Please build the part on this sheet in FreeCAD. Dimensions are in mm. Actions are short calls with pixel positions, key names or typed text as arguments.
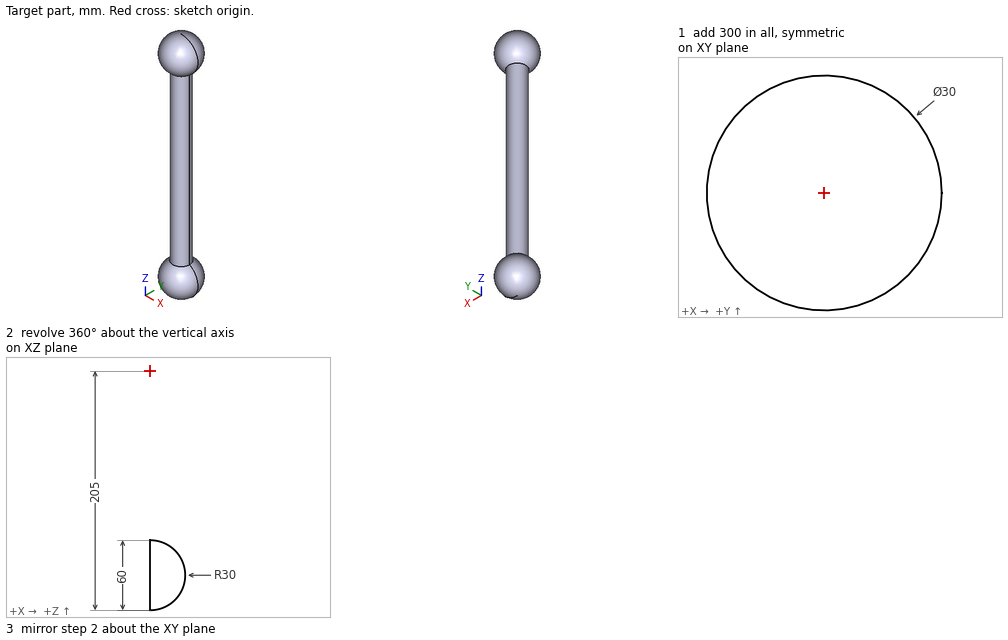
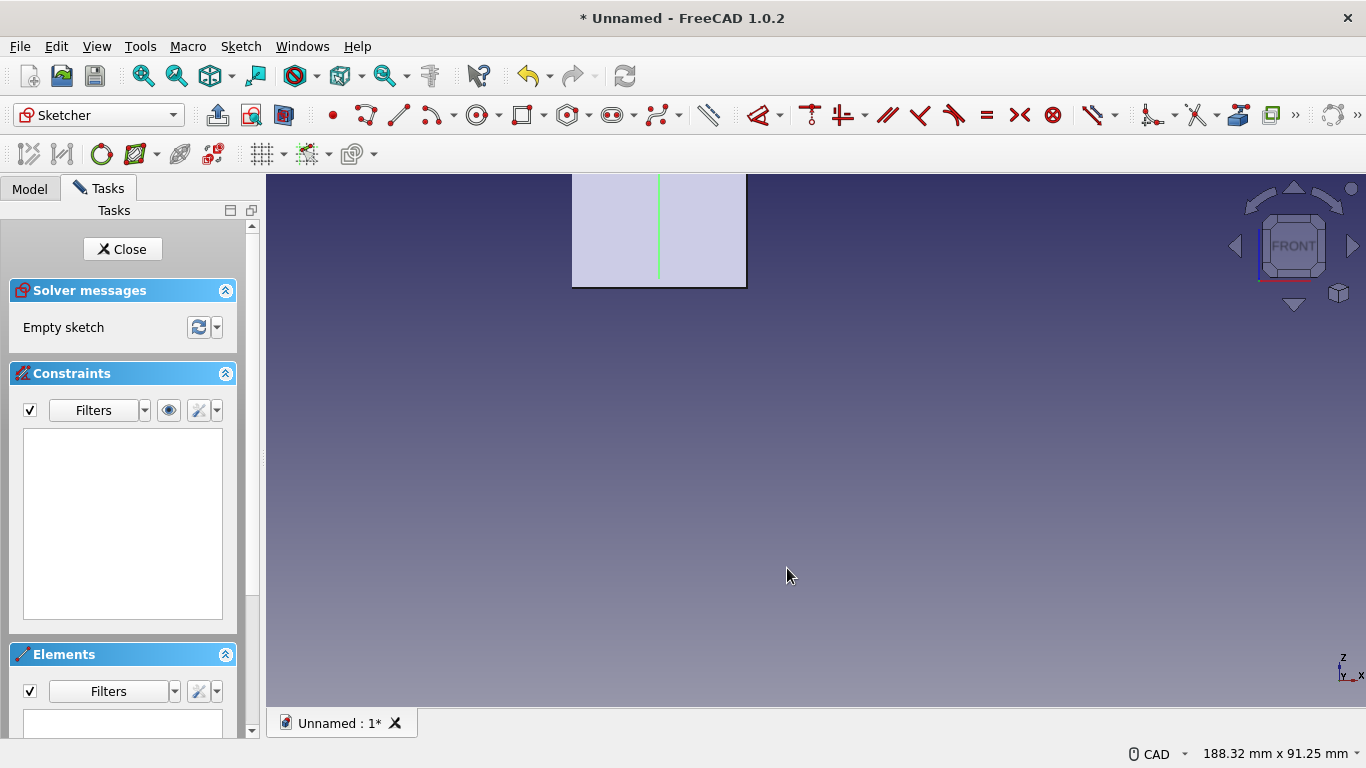
click(399, 116)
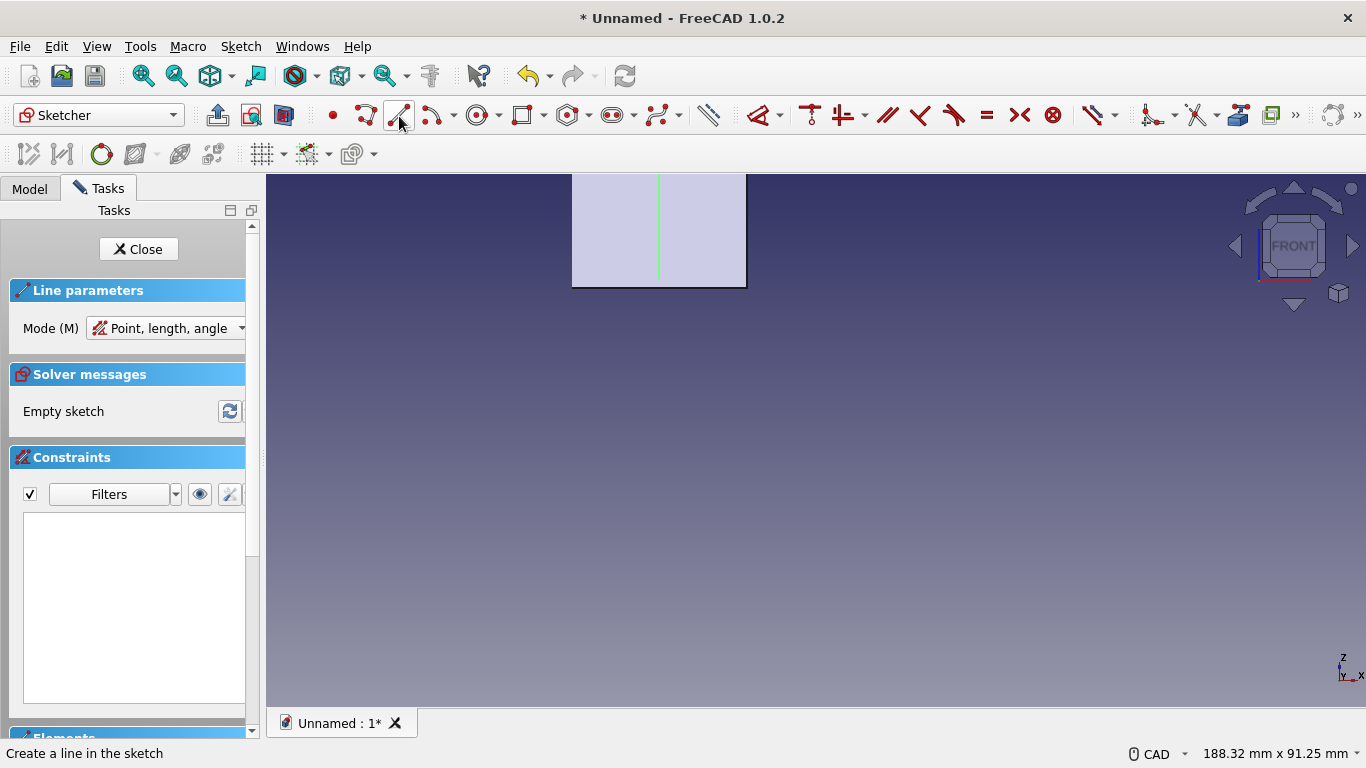
click(659, 609)
click(668, 258)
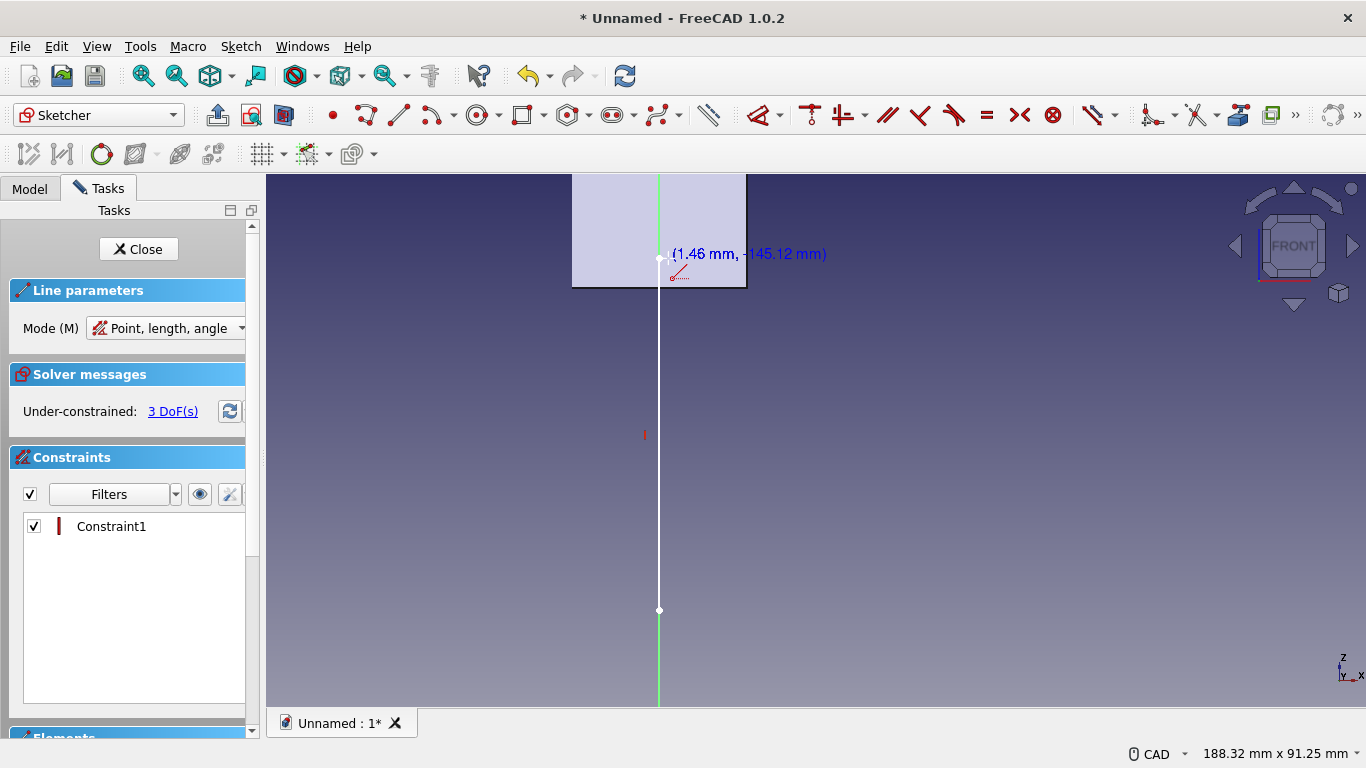
click(454, 116)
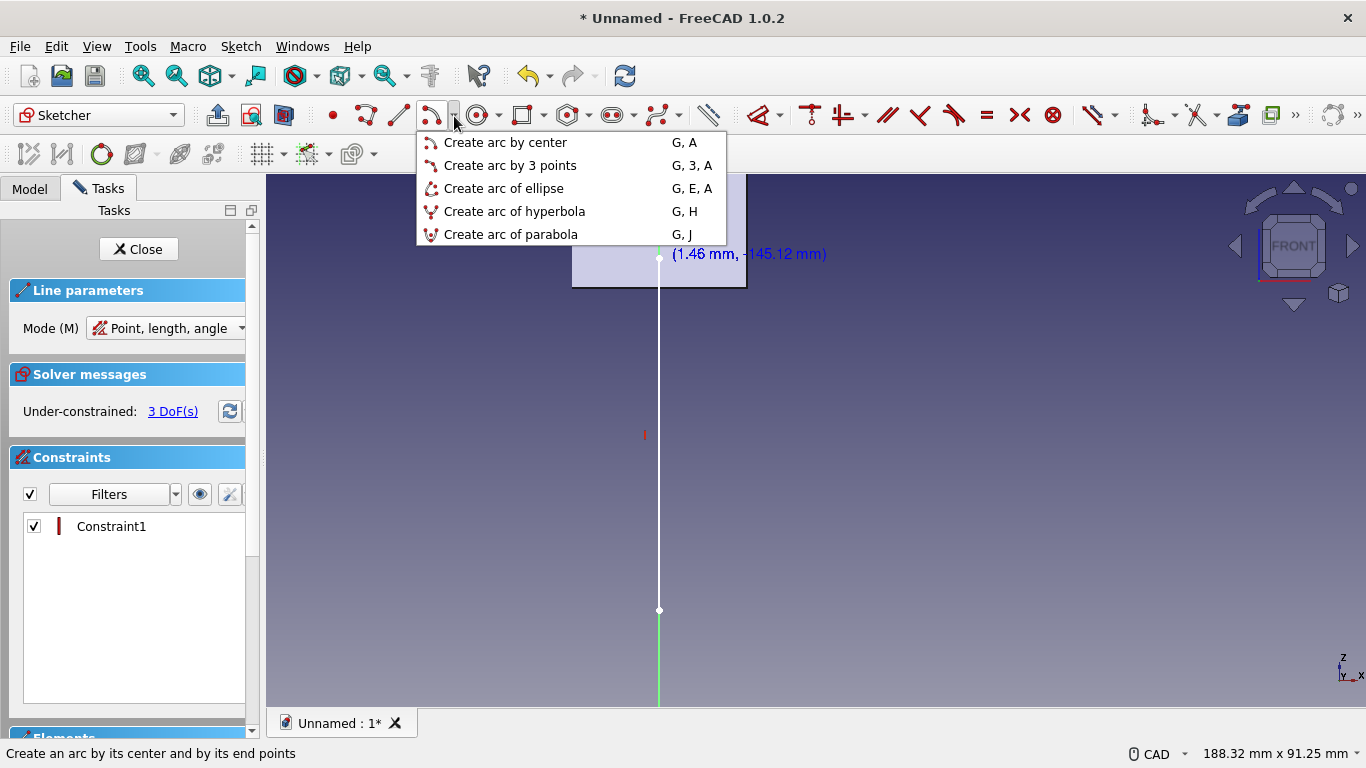
click(572, 166)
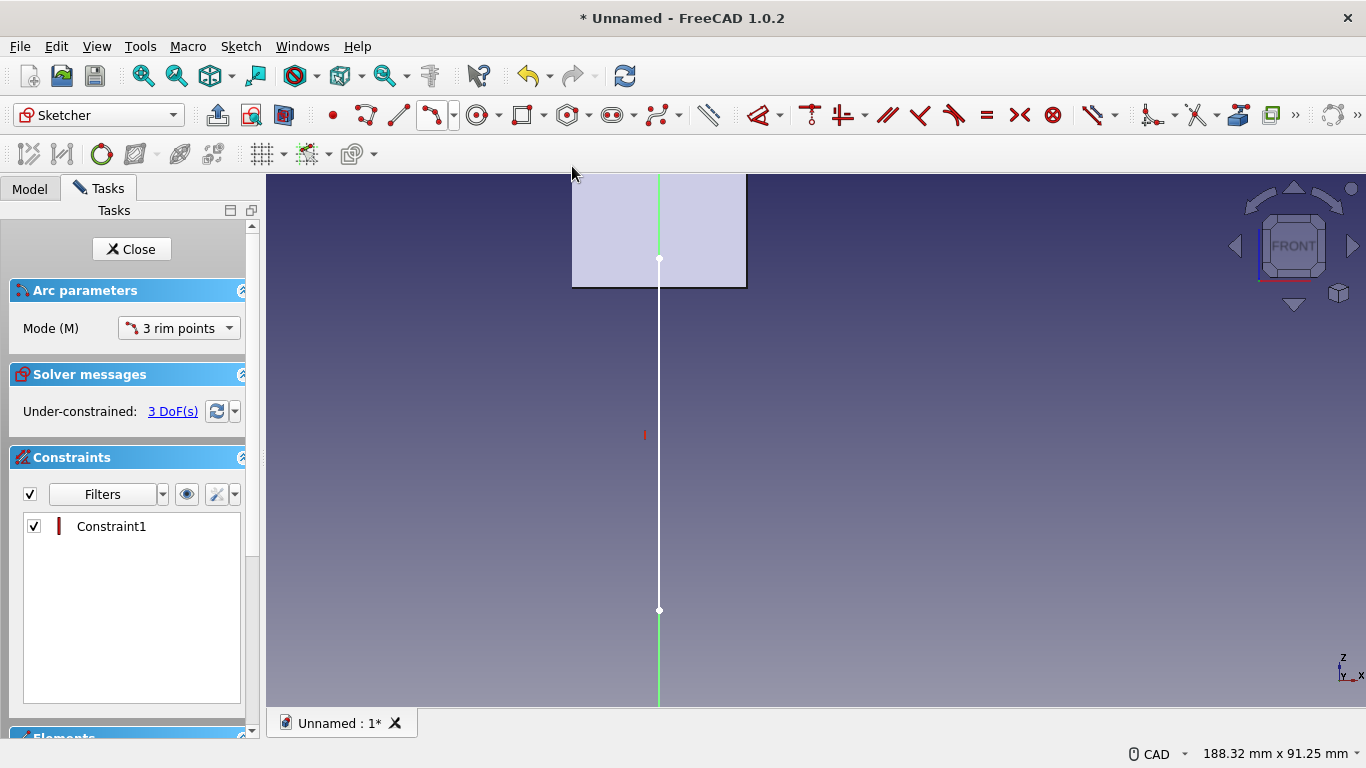
click(668, 258)
click(659, 610)
click(835, 434)
key(Escape)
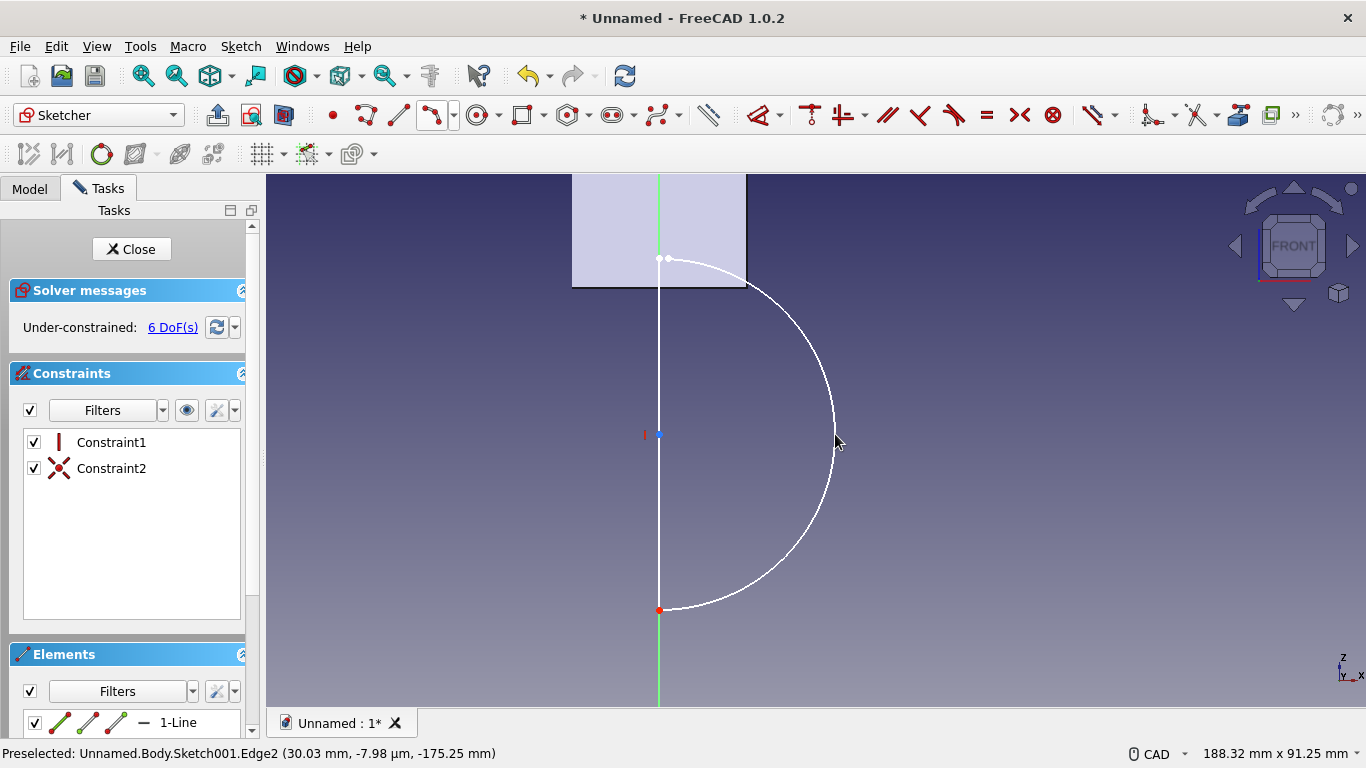
click(659, 434)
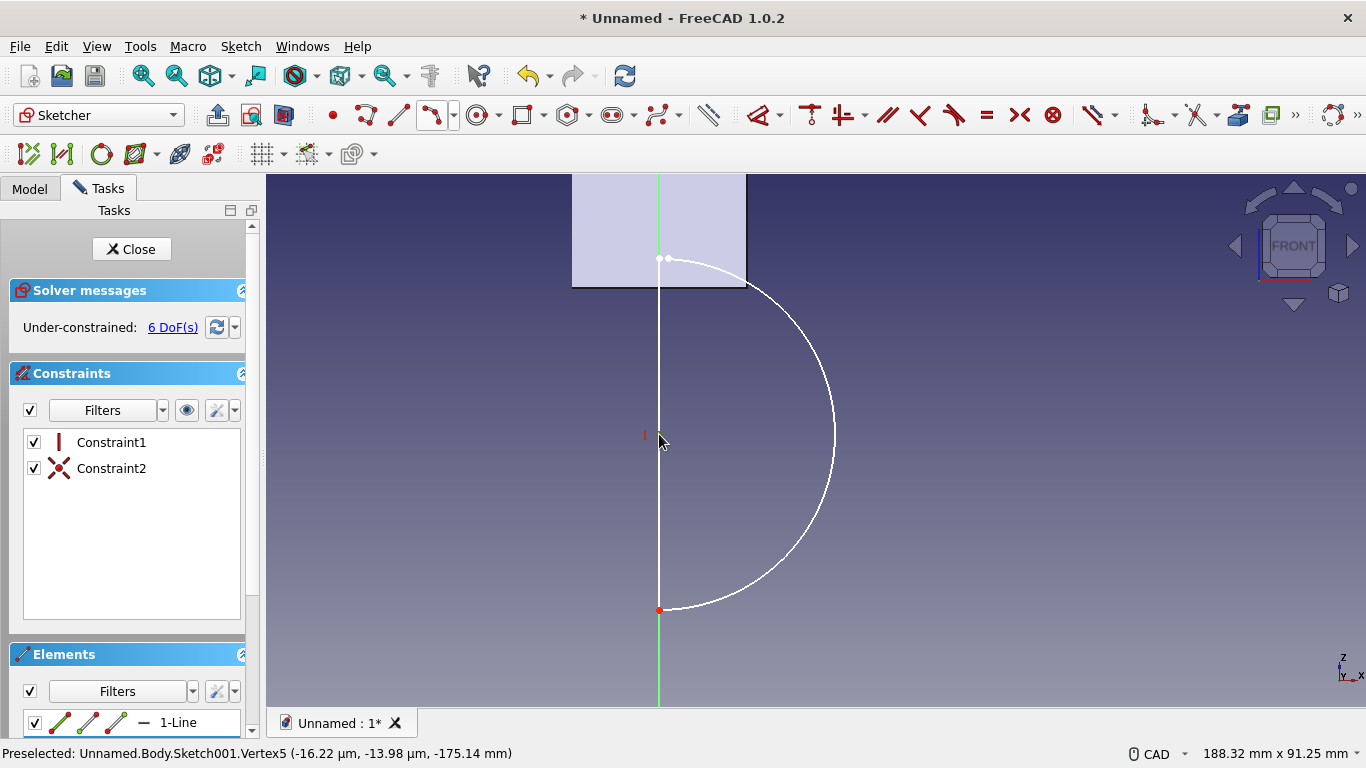
click(659, 645)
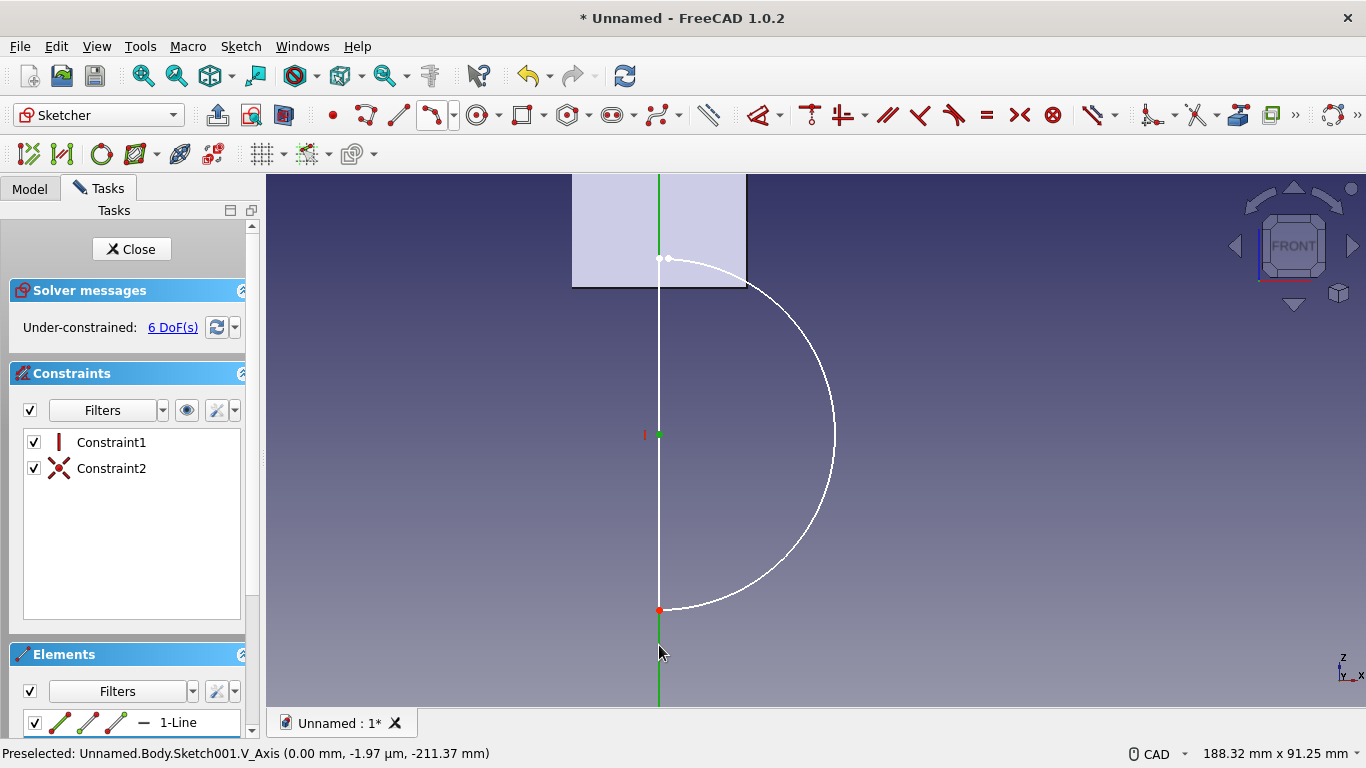
click(810, 116)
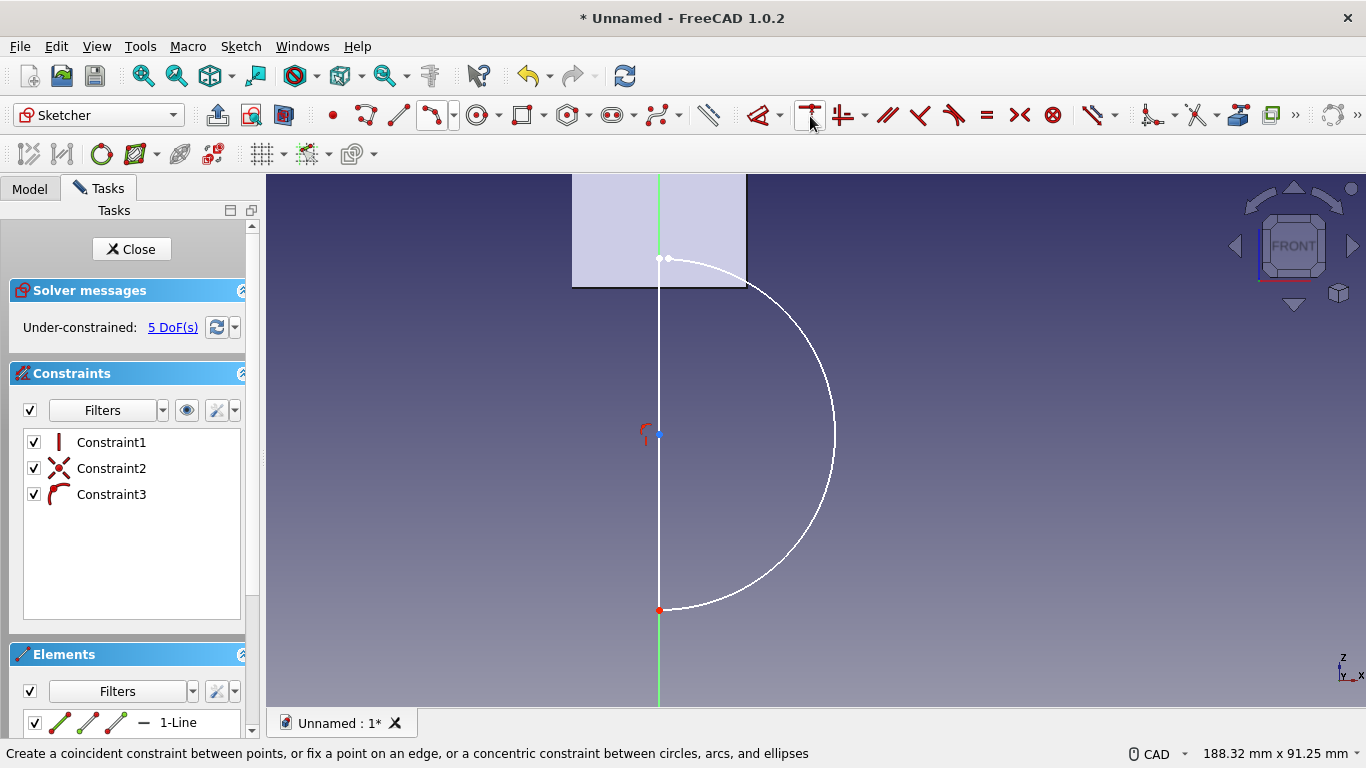
click(800, 540)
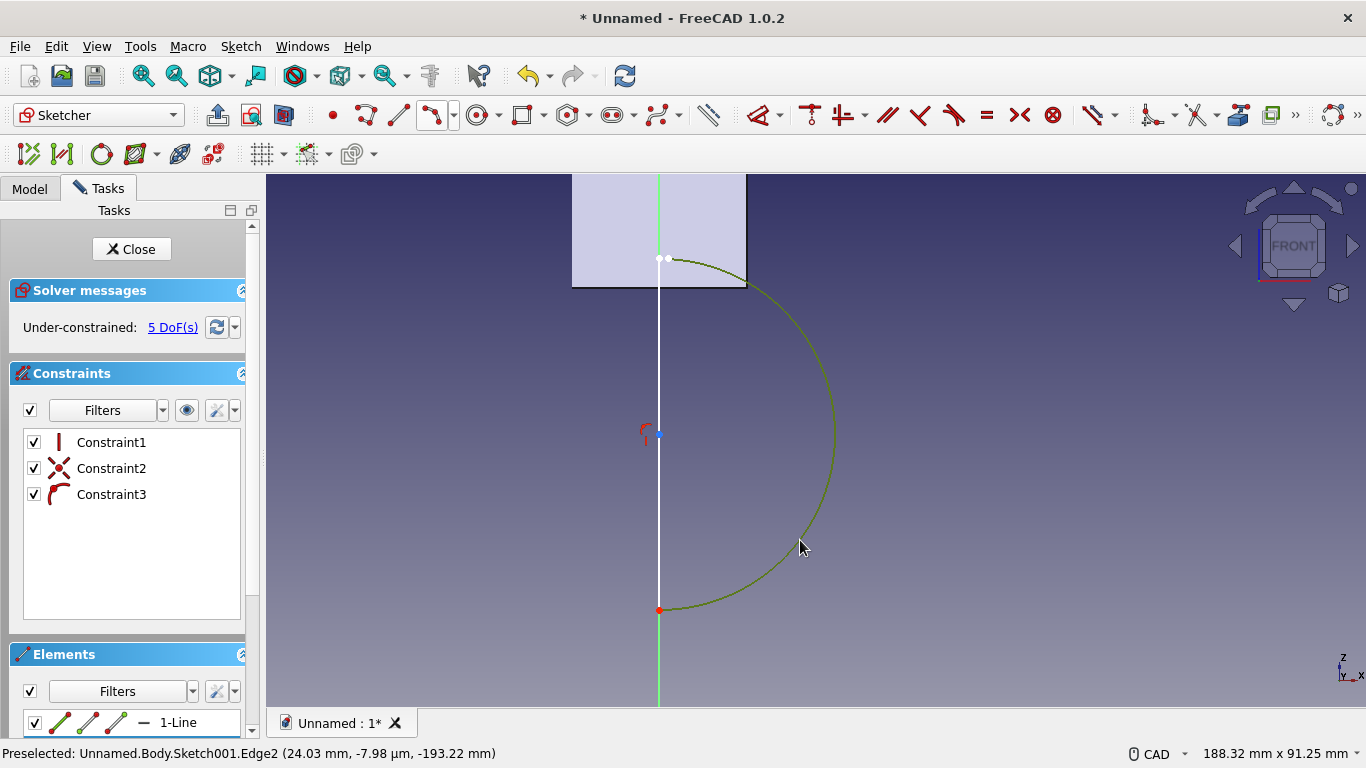
click(780, 116)